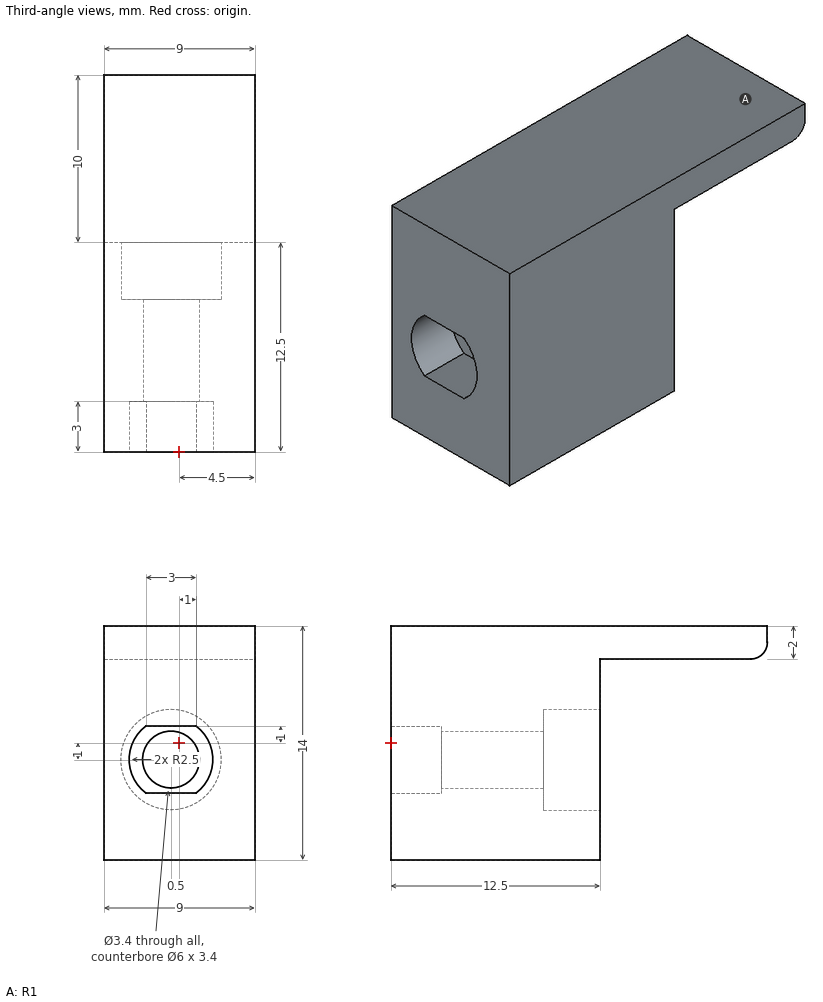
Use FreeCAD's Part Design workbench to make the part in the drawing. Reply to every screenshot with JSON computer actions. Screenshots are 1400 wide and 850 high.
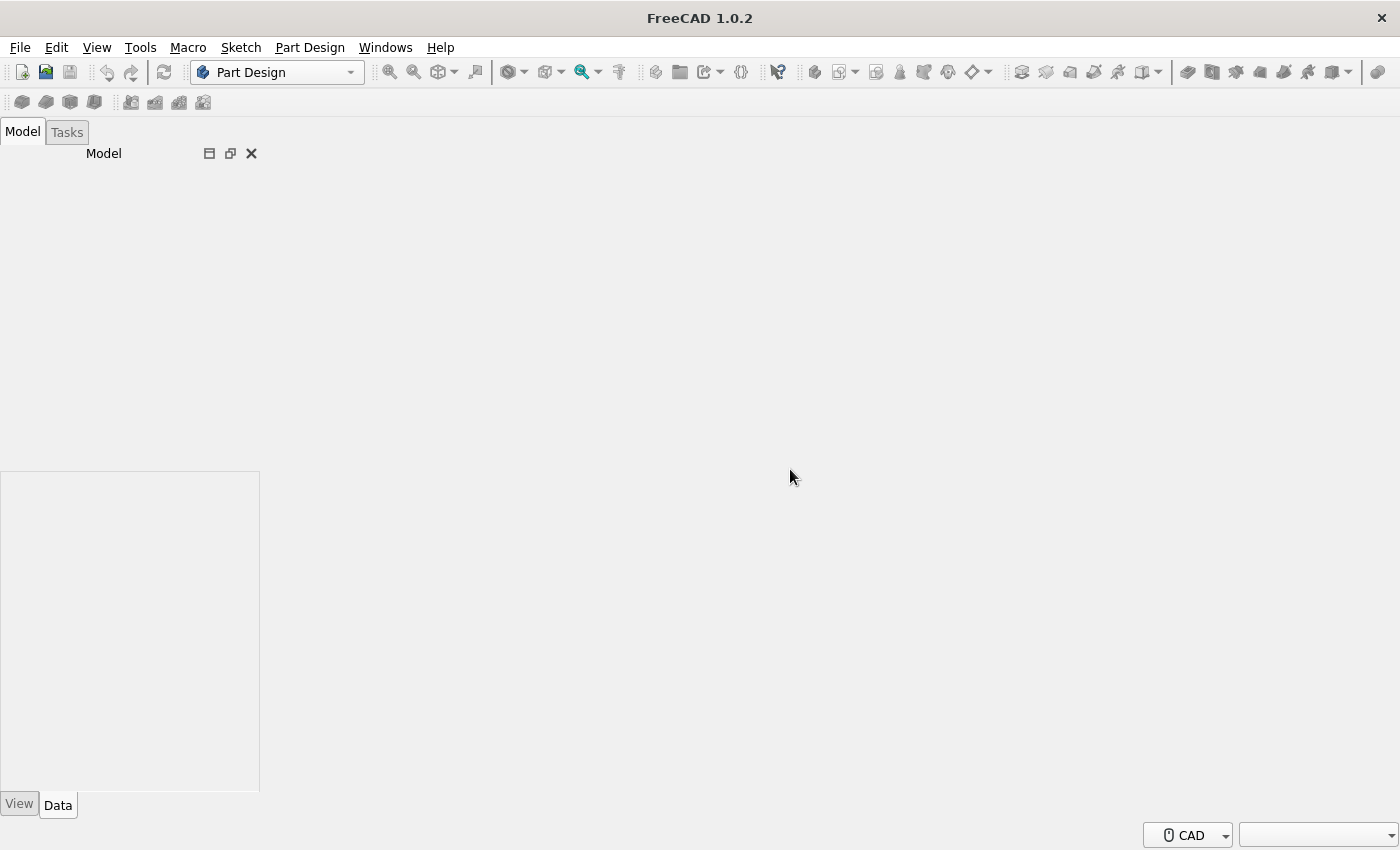
{"action": "left_click", "coordinate": [22, 72]}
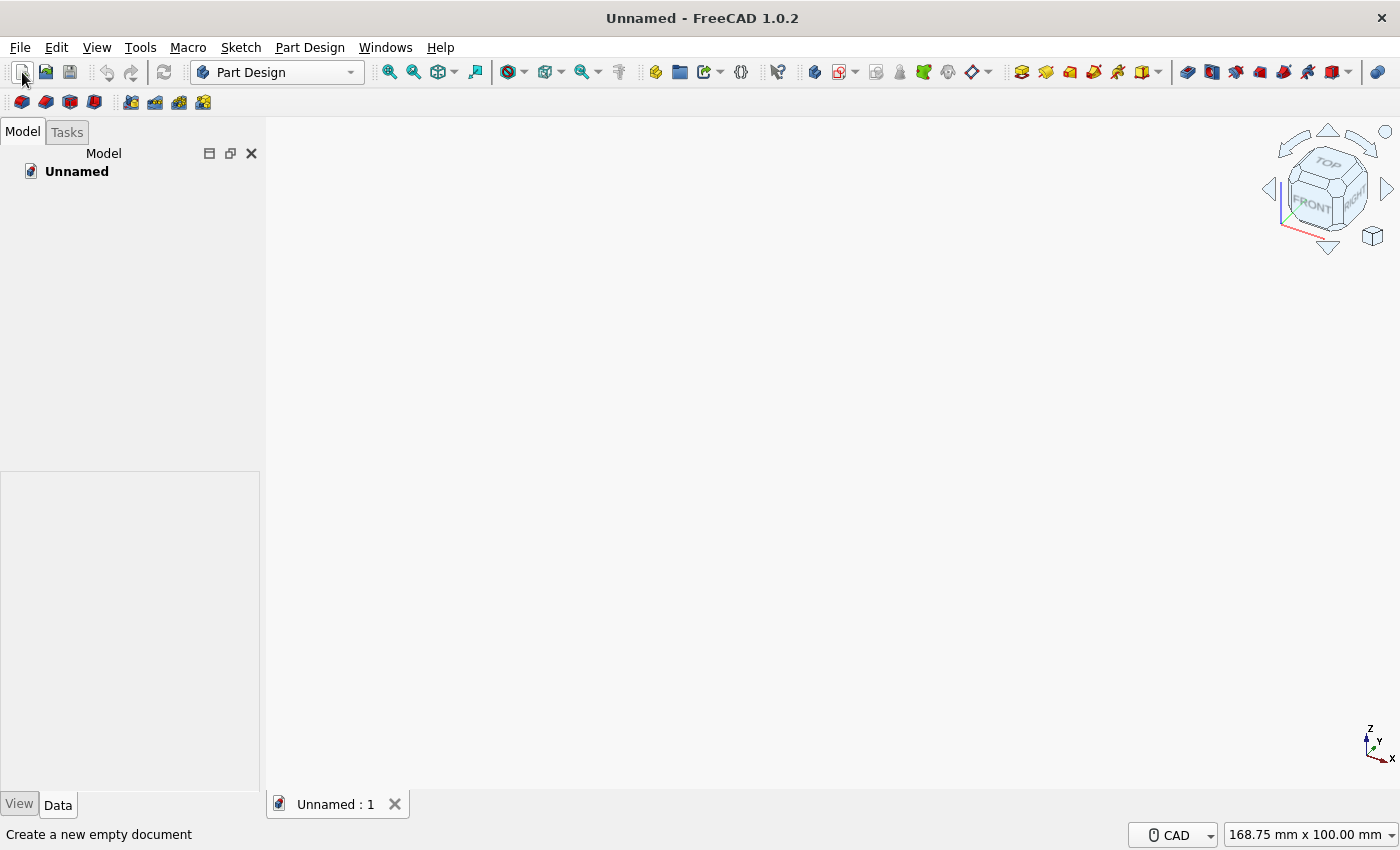
{"action": "left_click", "coordinate": [840, 72]}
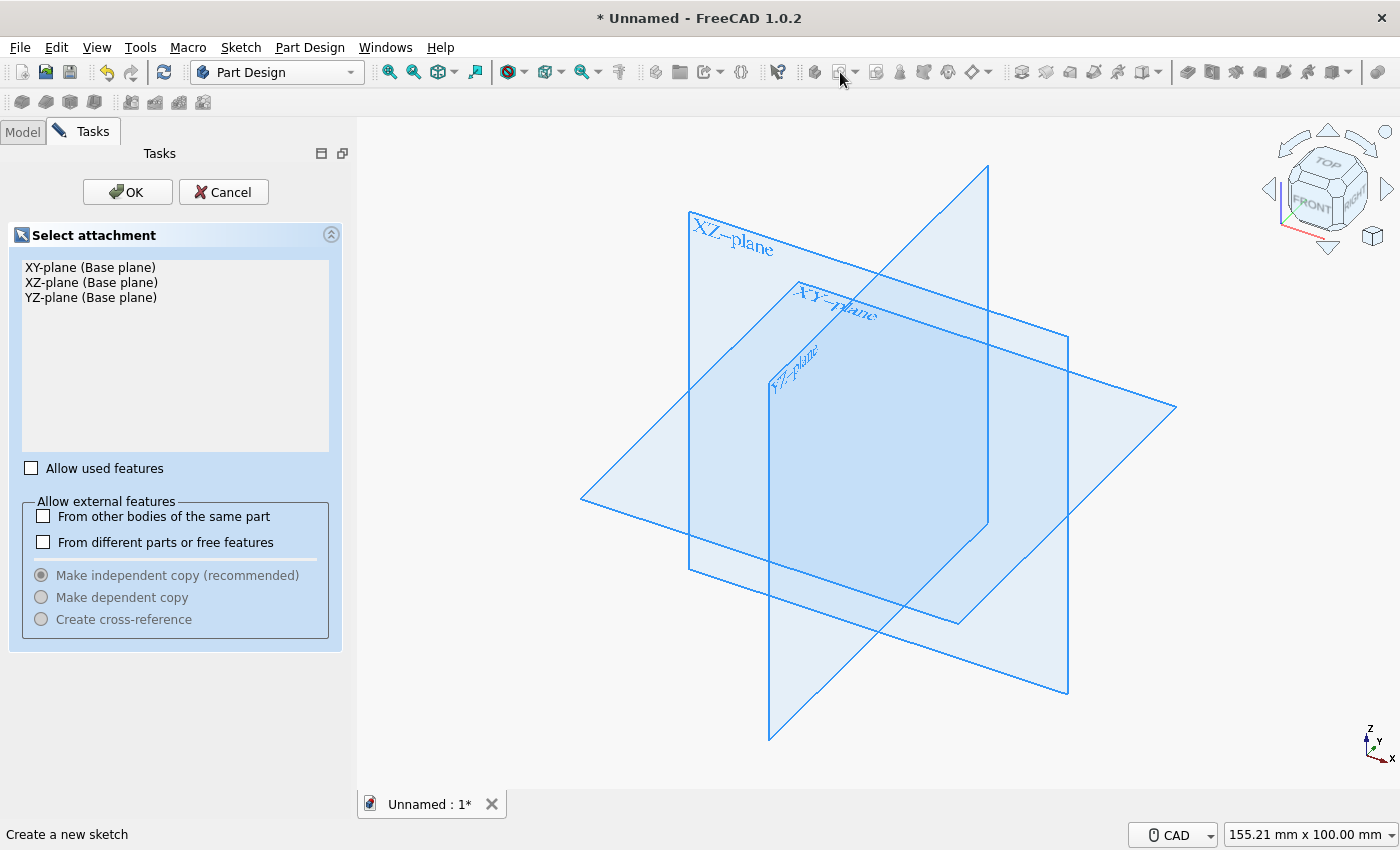
{"action": "left_click", "coordinate": [82, 282]}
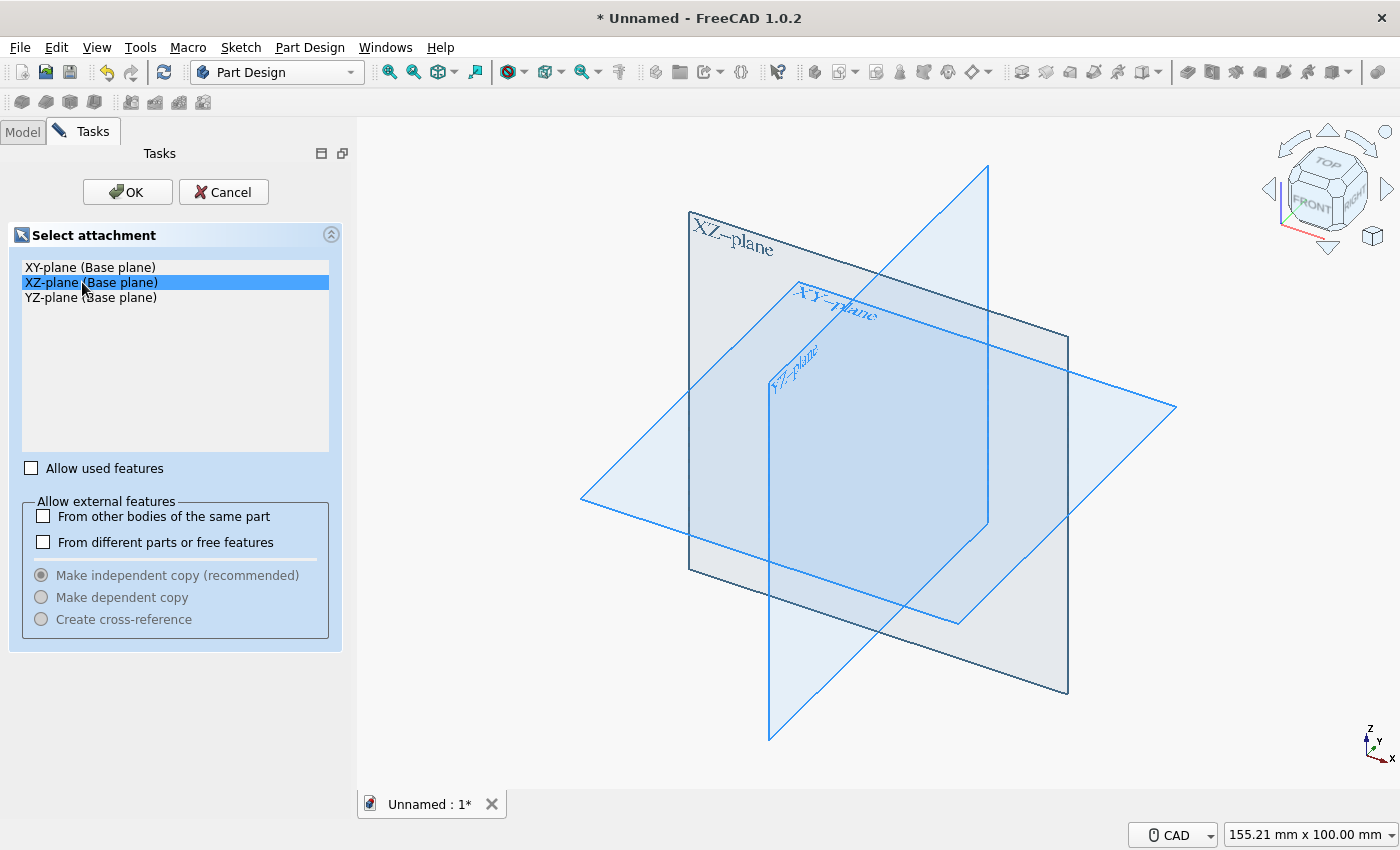
{"action": "left_click", "coordinate": [128, 192]}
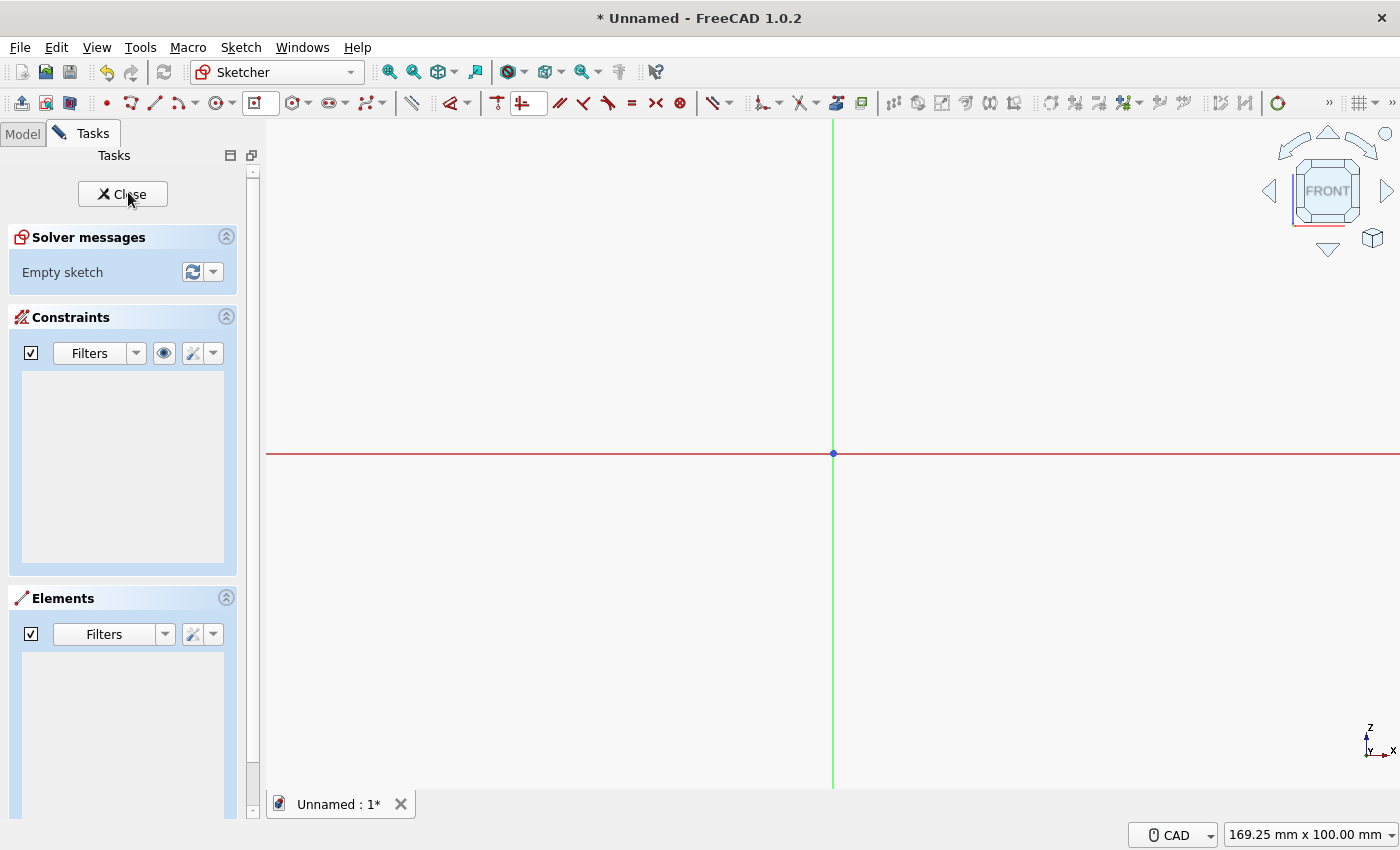
{"action": "scroll", "coordinate": [850, 454], "scroll_direction": "up", "scroll_amount": 8}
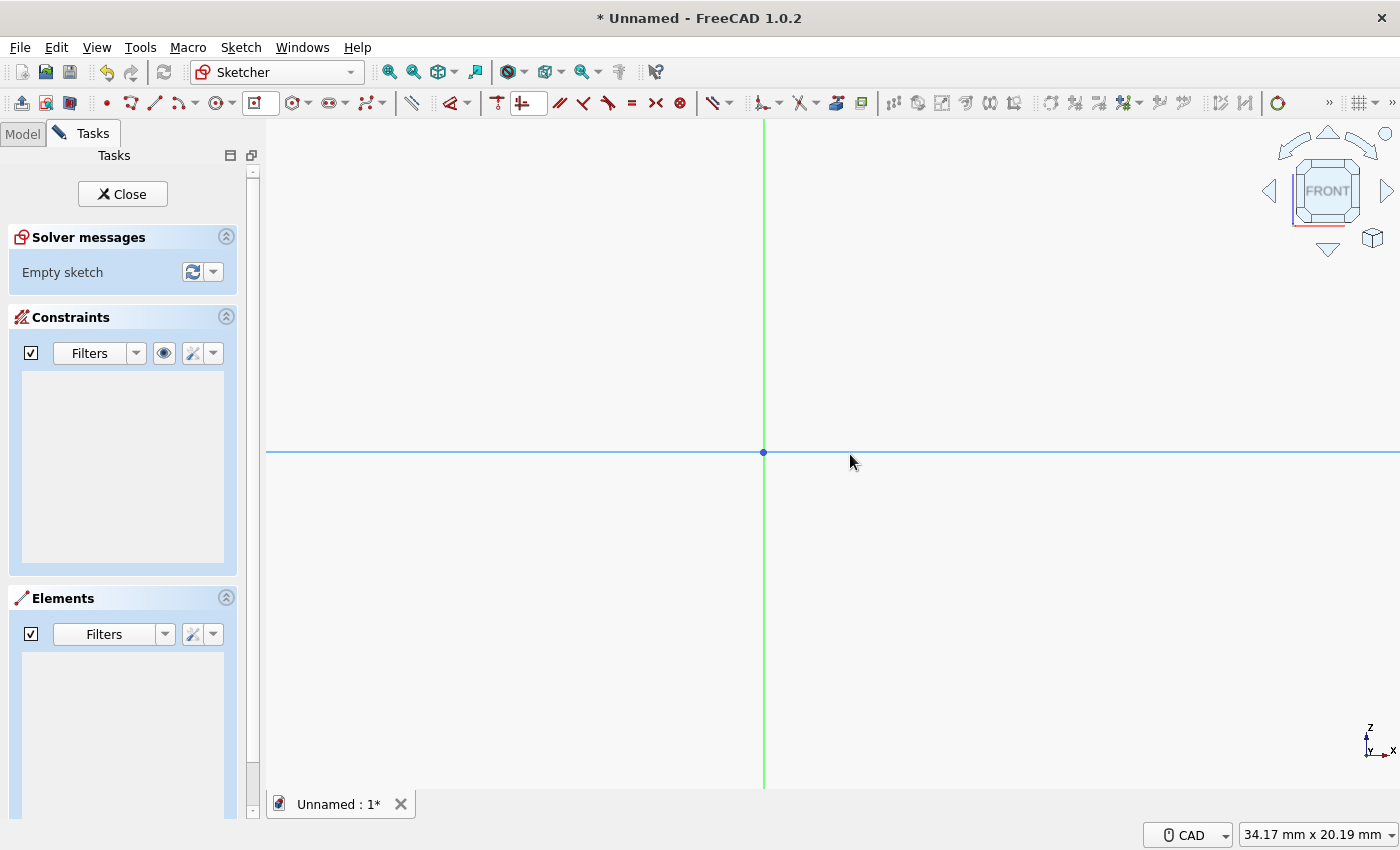
{"action": "key", "text": "g v"}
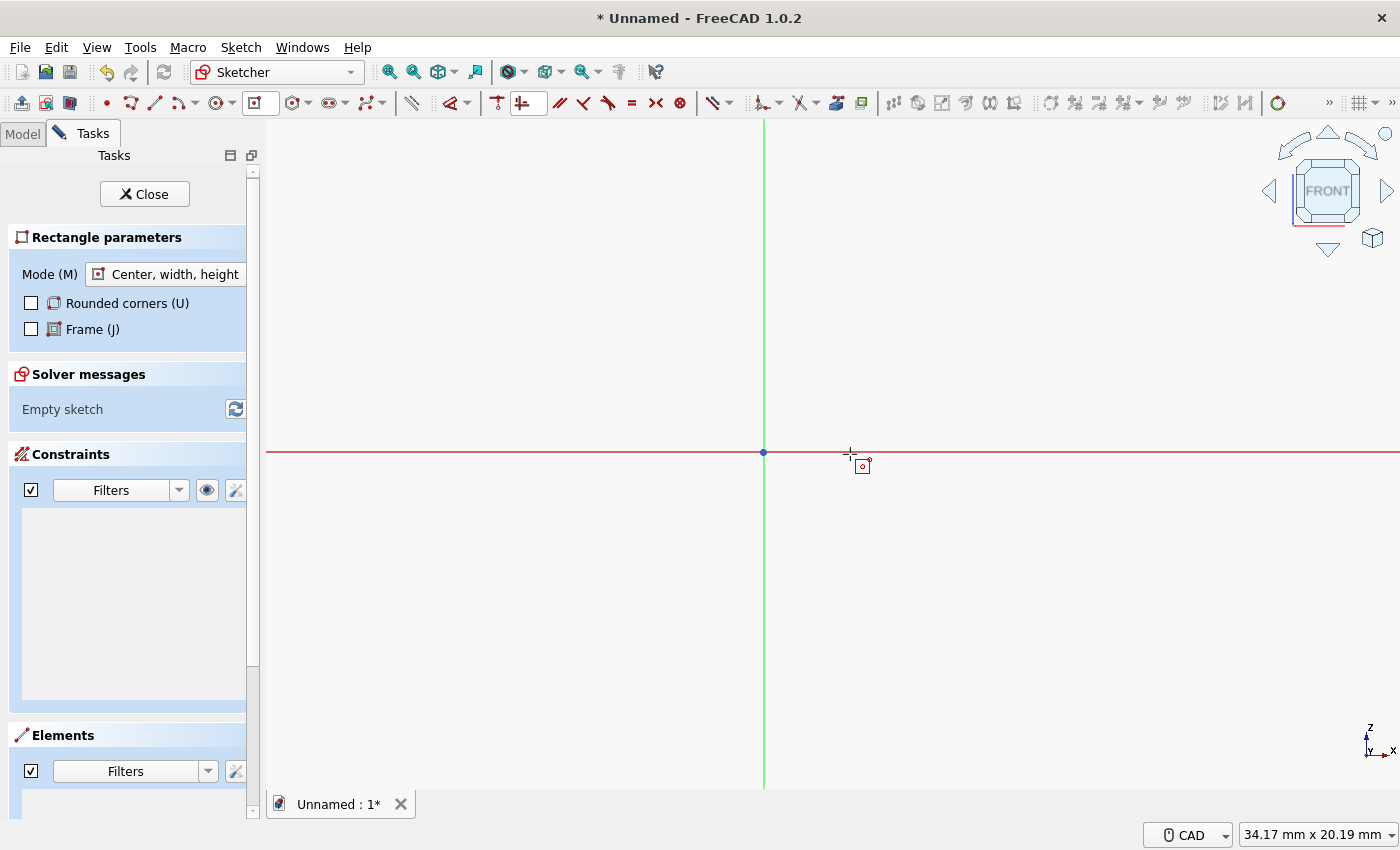
{"action": "left_click", "coordinate": [764, 452]}
{"action": "mouse_move", "coordinate": [913, 220]}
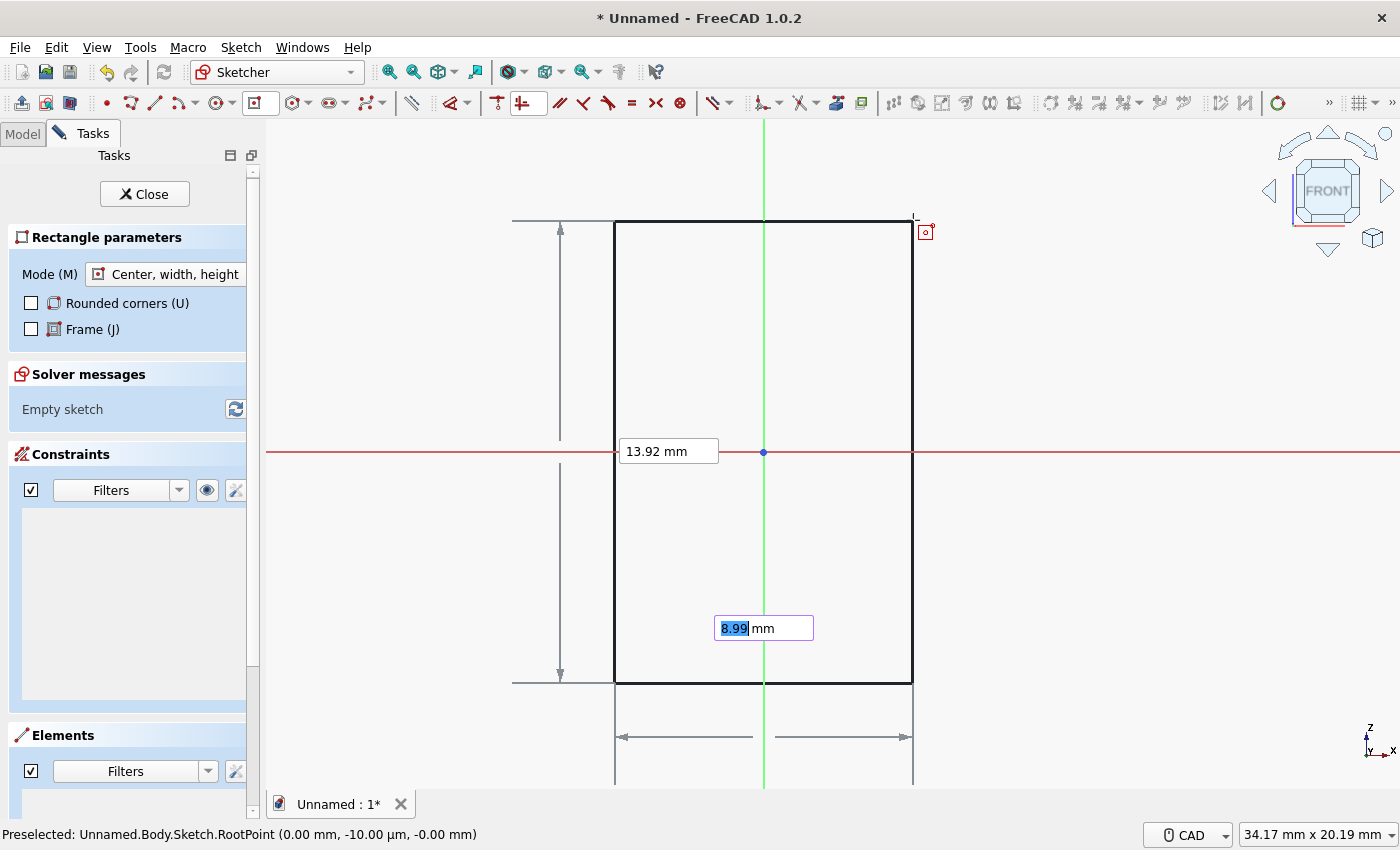
{"action": "type", "text": "9"}
{"action": "key", "text": "Tab"}
{"action": "type", "text": "14"}
{"action": "key", "text": "Return"}
{"action": "key", "text": "Escape"}